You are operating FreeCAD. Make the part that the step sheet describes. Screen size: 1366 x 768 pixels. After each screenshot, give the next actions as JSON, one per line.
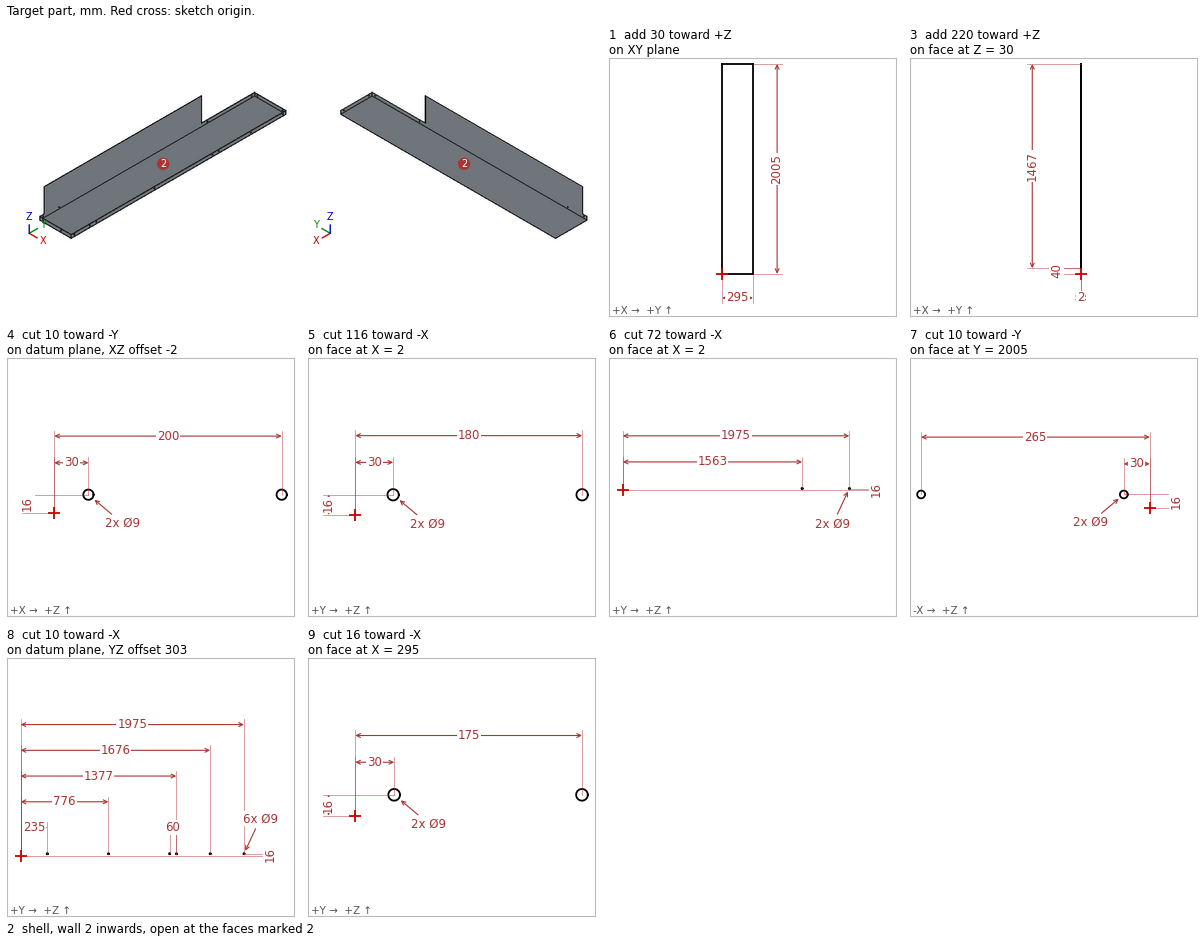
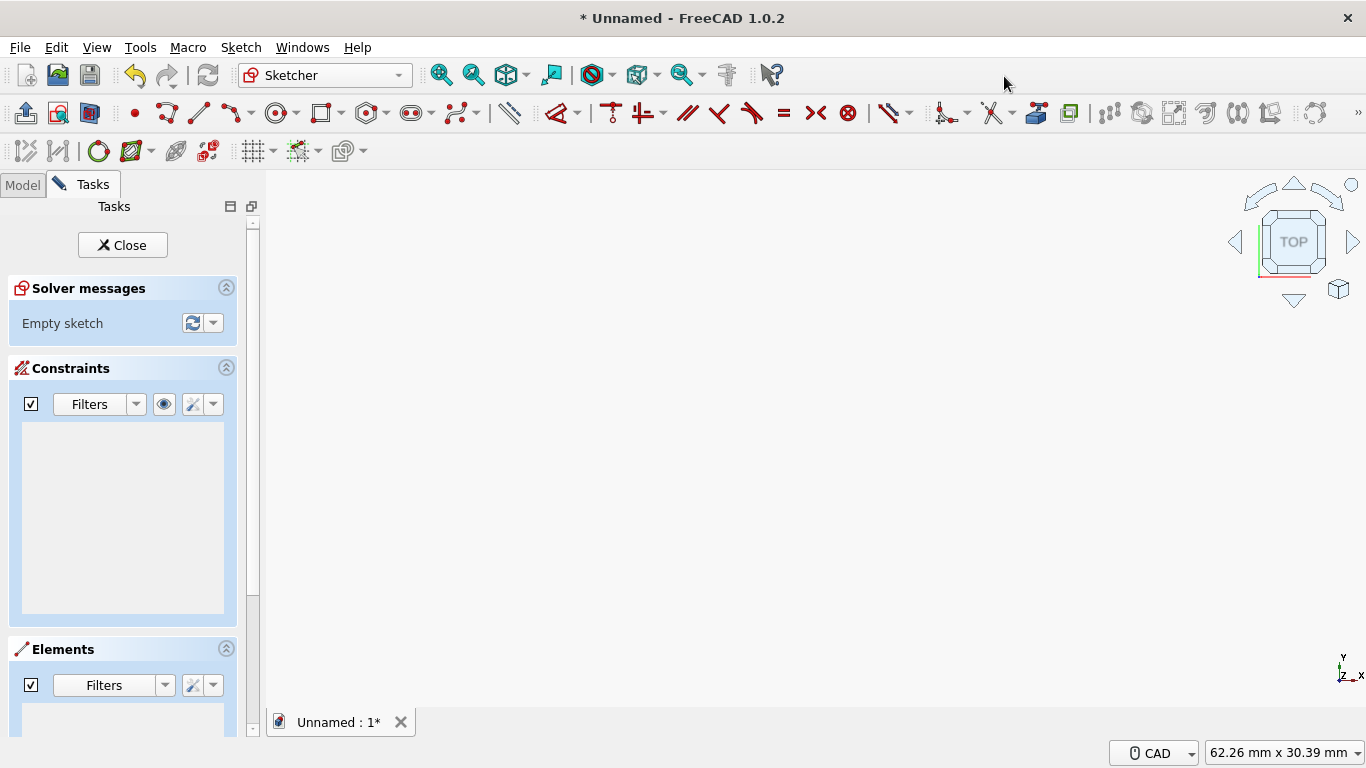
{"action": "scroll", "coordinate": [748, 438], "scroll_direction": "down", "scroll_amount": 15}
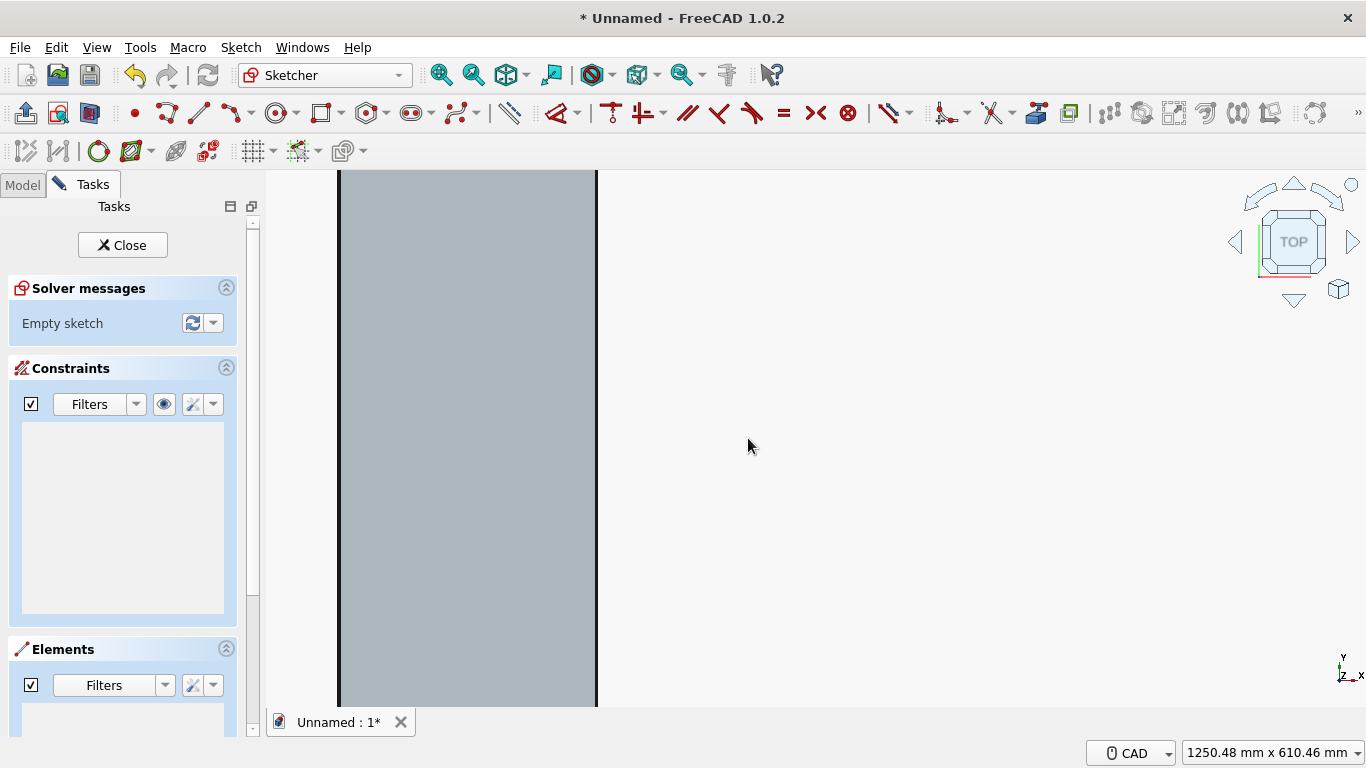
{"action": "scroll", "coordinate": [881, 220], "scroll_direction": "down", "scroll_amount": 7}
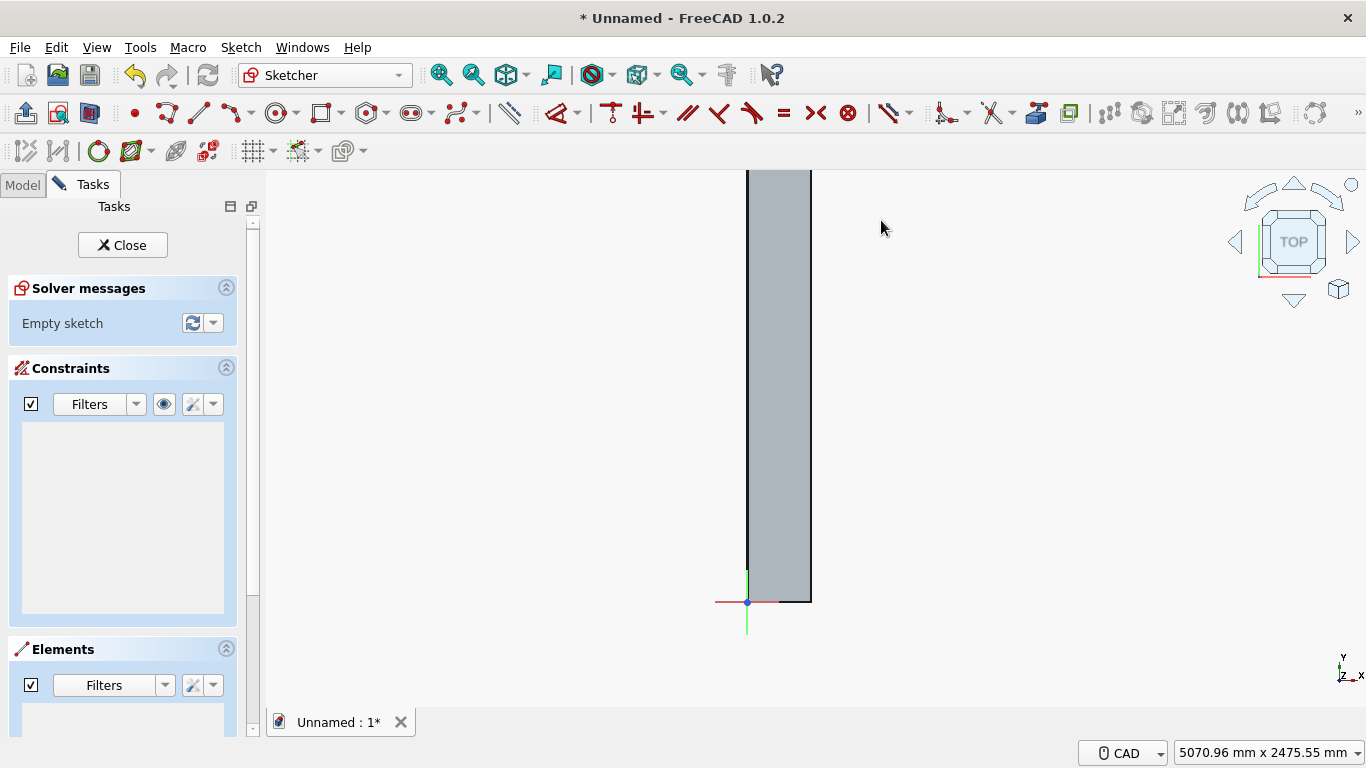
{"action": "left_click", "coordinate": [322, 114]}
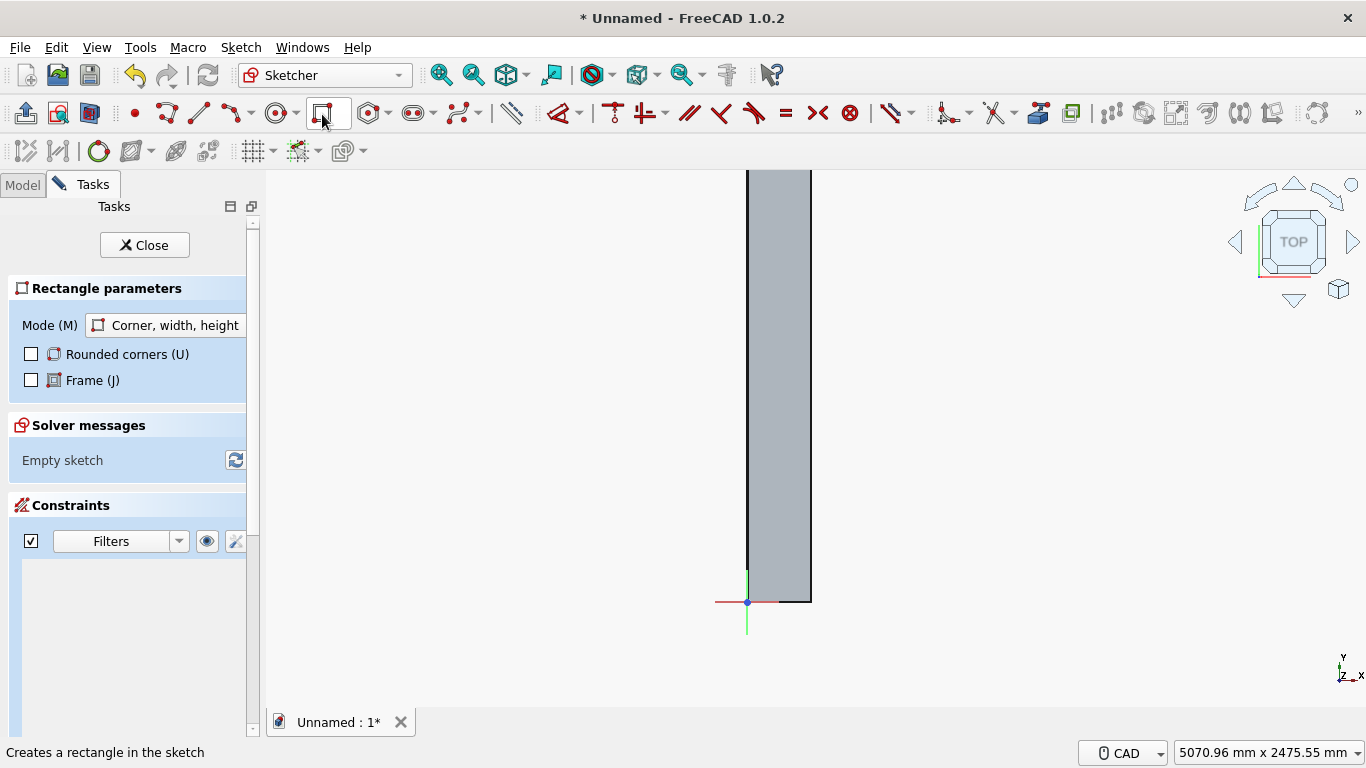
{"action": "scroll", "coordinate": [747, 275], "scroll_direction": "up", "scroll_amount": 19}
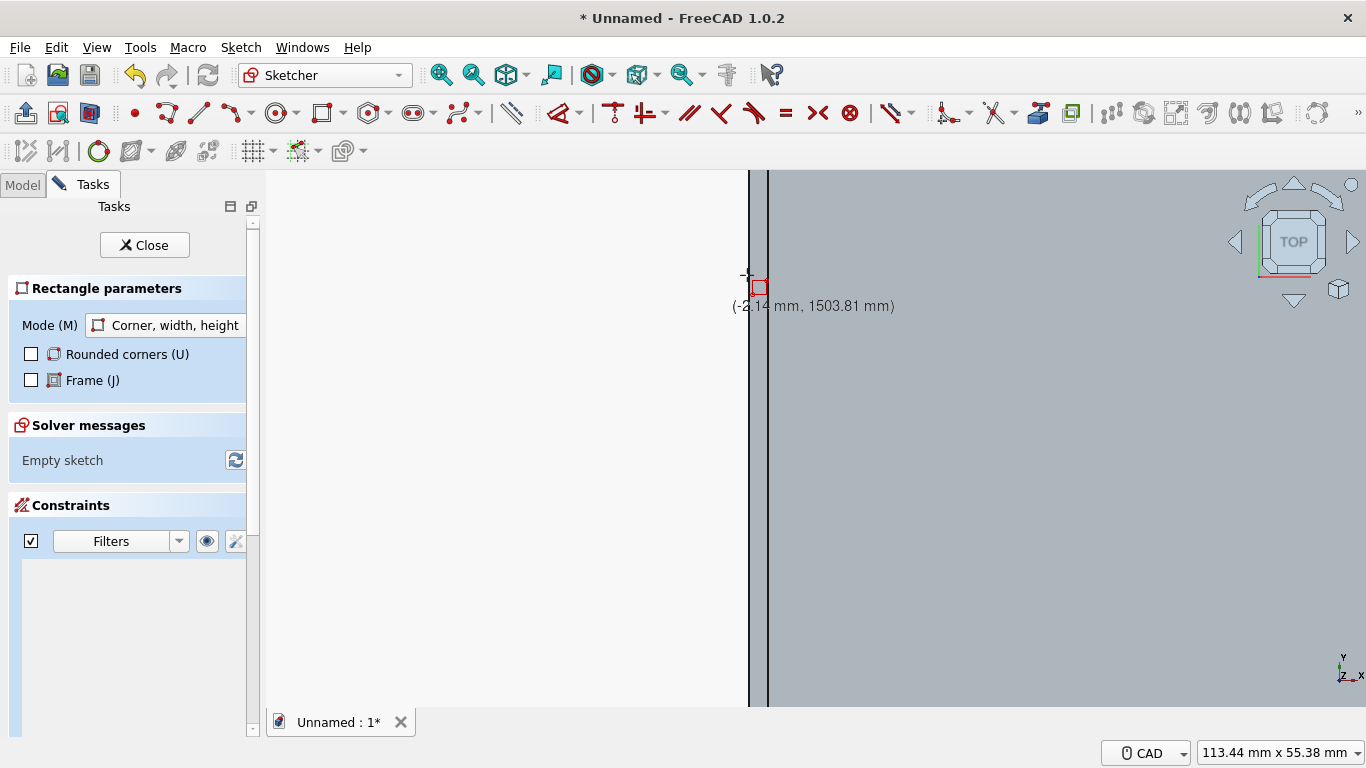
{"action": "scroll", "coordinate": [747, 238], "scroll_direction": "down", "scroll_amount": 18}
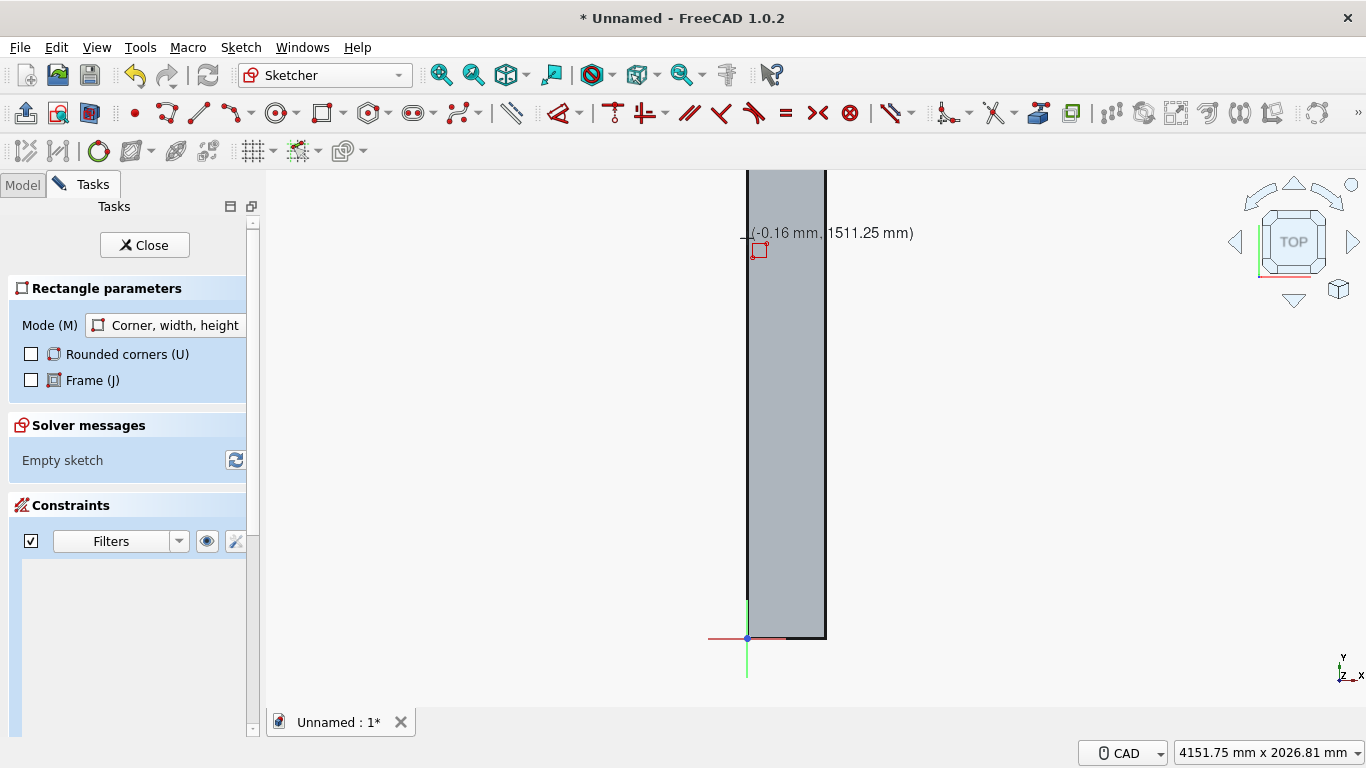
{"action": "left_click", "coordinate": [747, 239]}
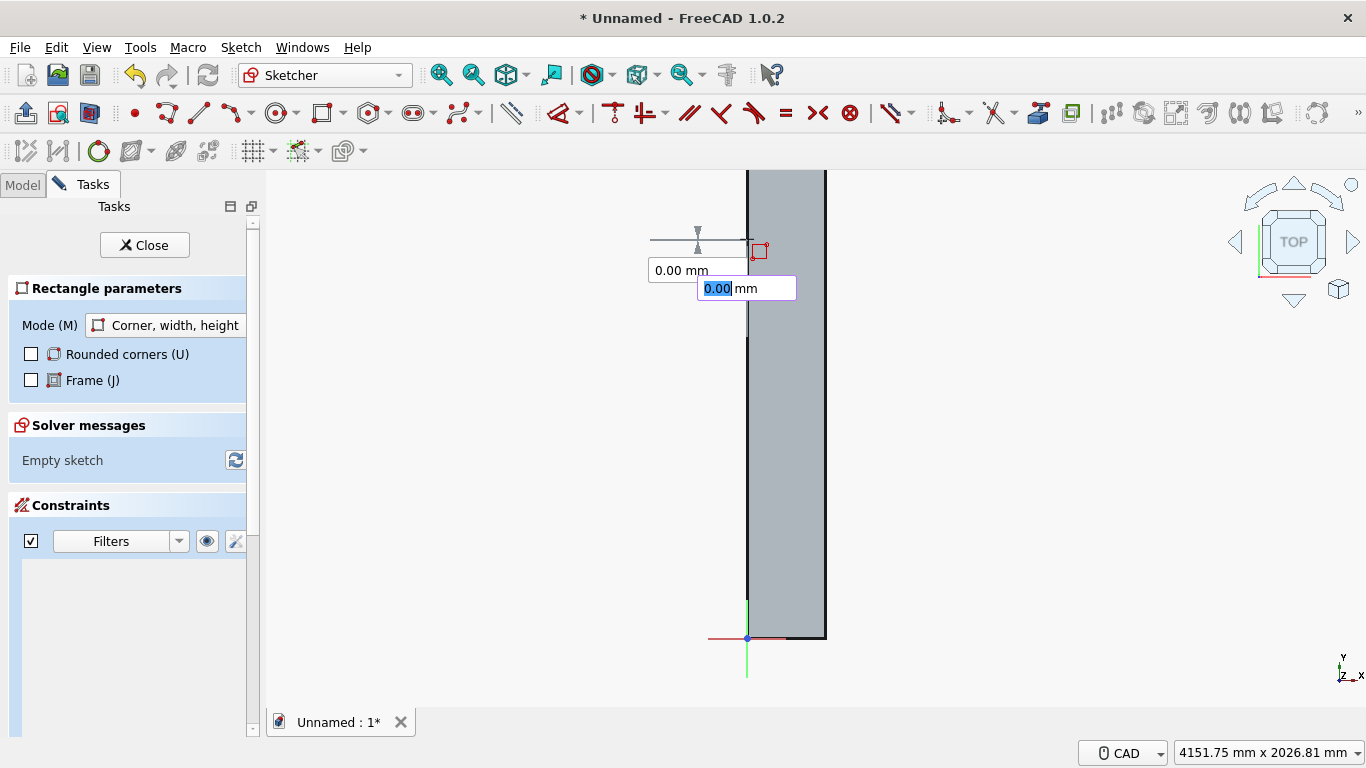
{"action": "scroll", "coordinate": [748, 628], "scroll_direction": "up", "scroll_amount": 18}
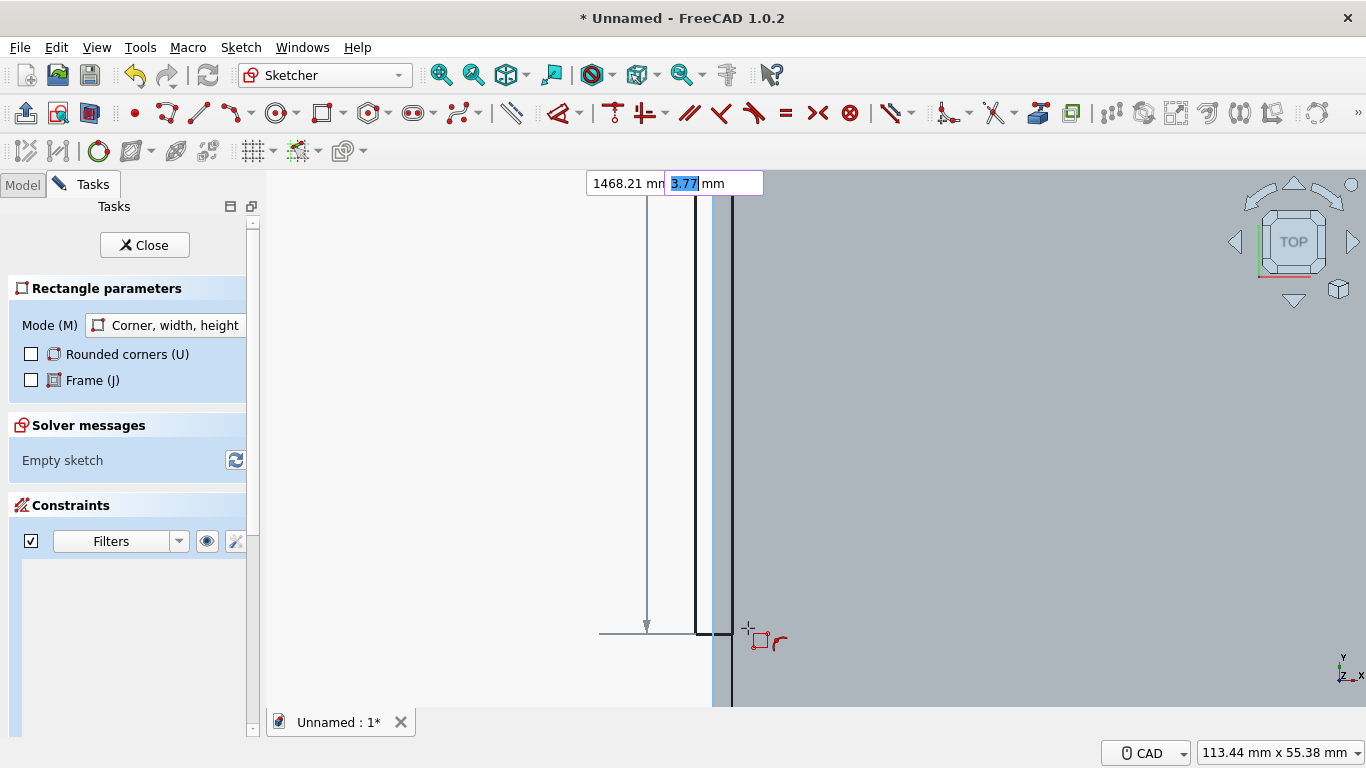
{"action": "left_click", "coordinate": [732, 596]}
{"action": "key", "text": "Escape"}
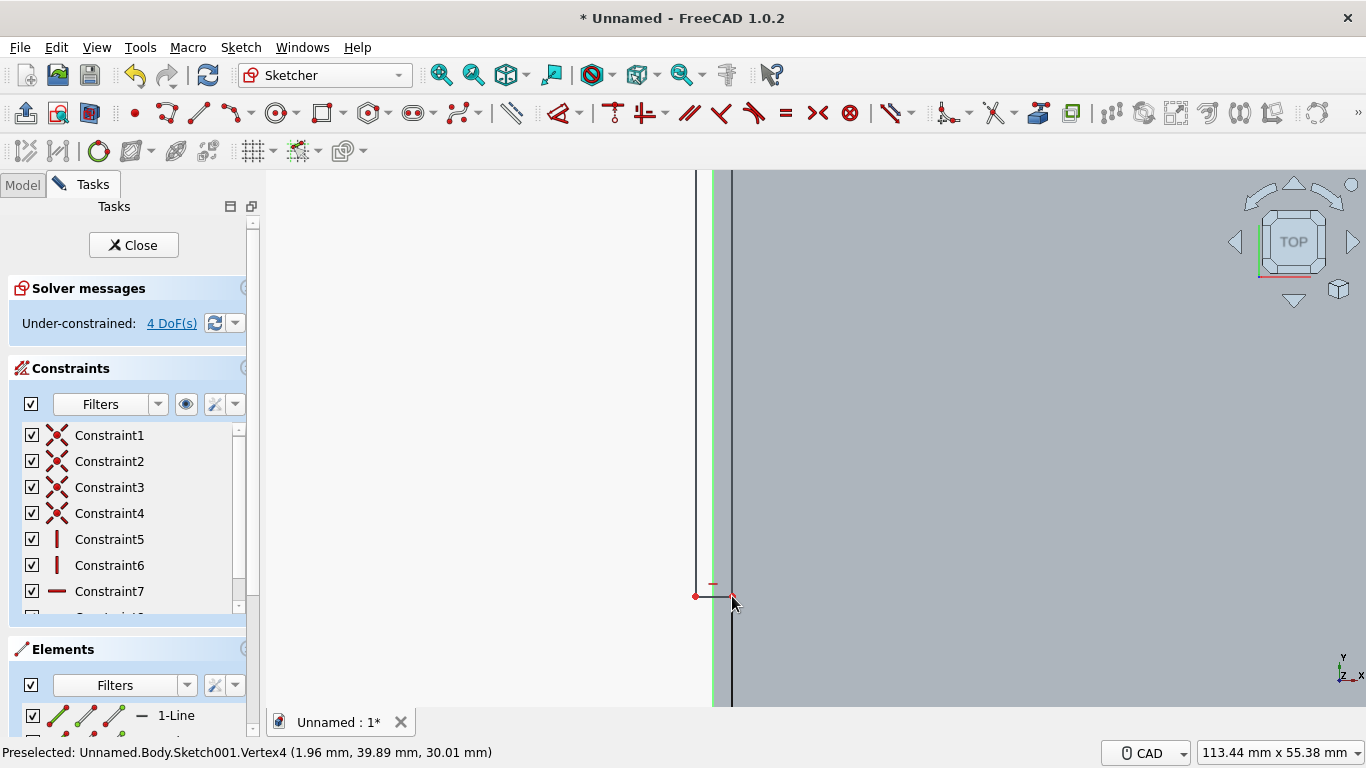
{"action": "scroll", "coordinate": [748, 628], "scroll_direction": "down", "scroll_amount": 18}